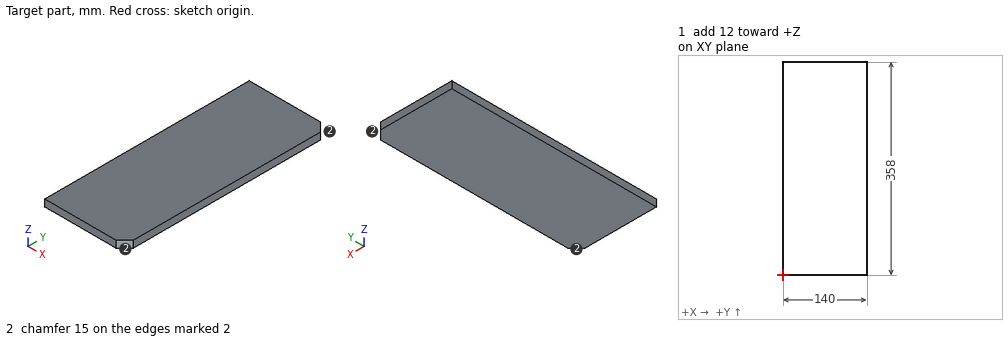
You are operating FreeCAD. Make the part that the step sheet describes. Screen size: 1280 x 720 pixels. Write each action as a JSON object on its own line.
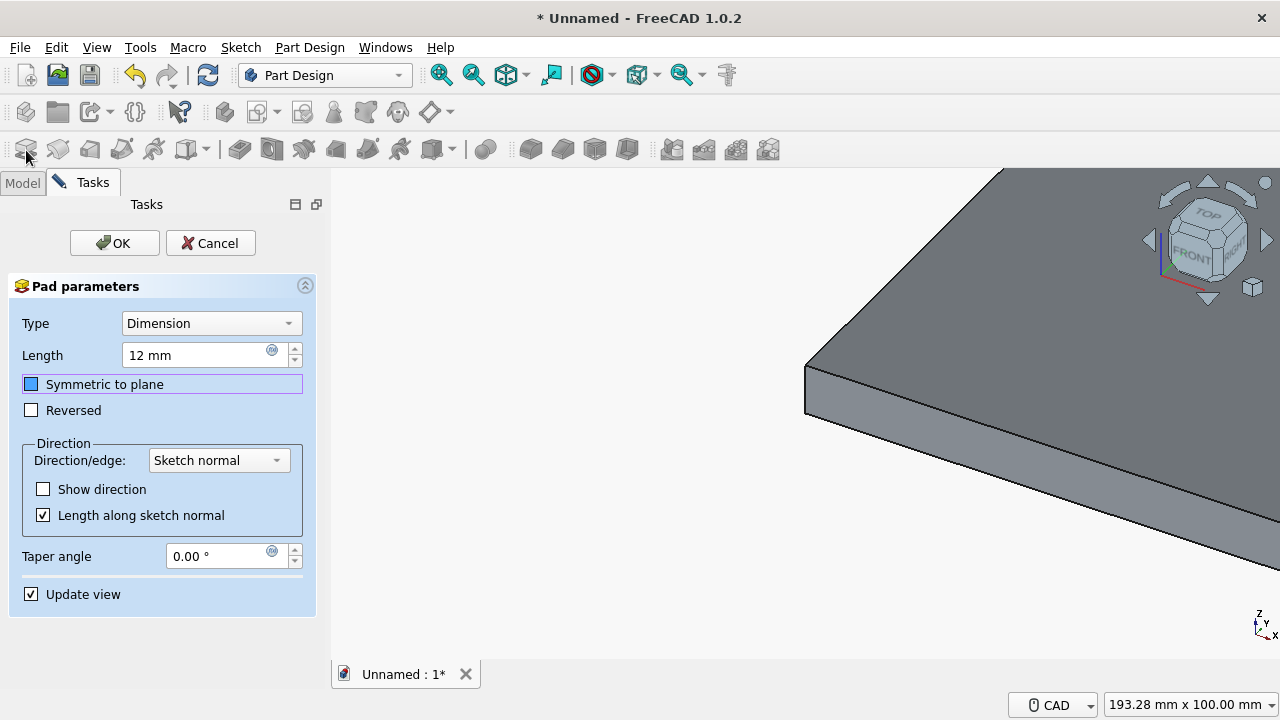
{"action": "left_click", "coordinate": [115, 243]}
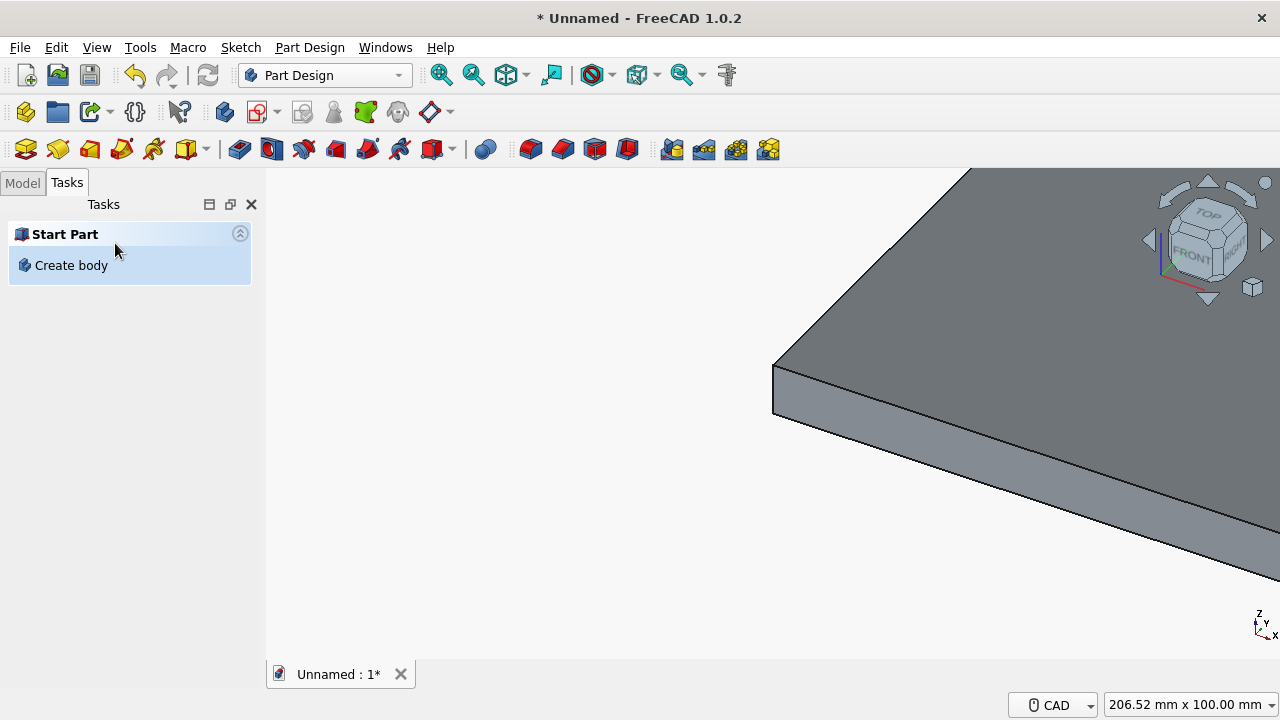
{"action": "left_click", "coordinate": [442, 76]}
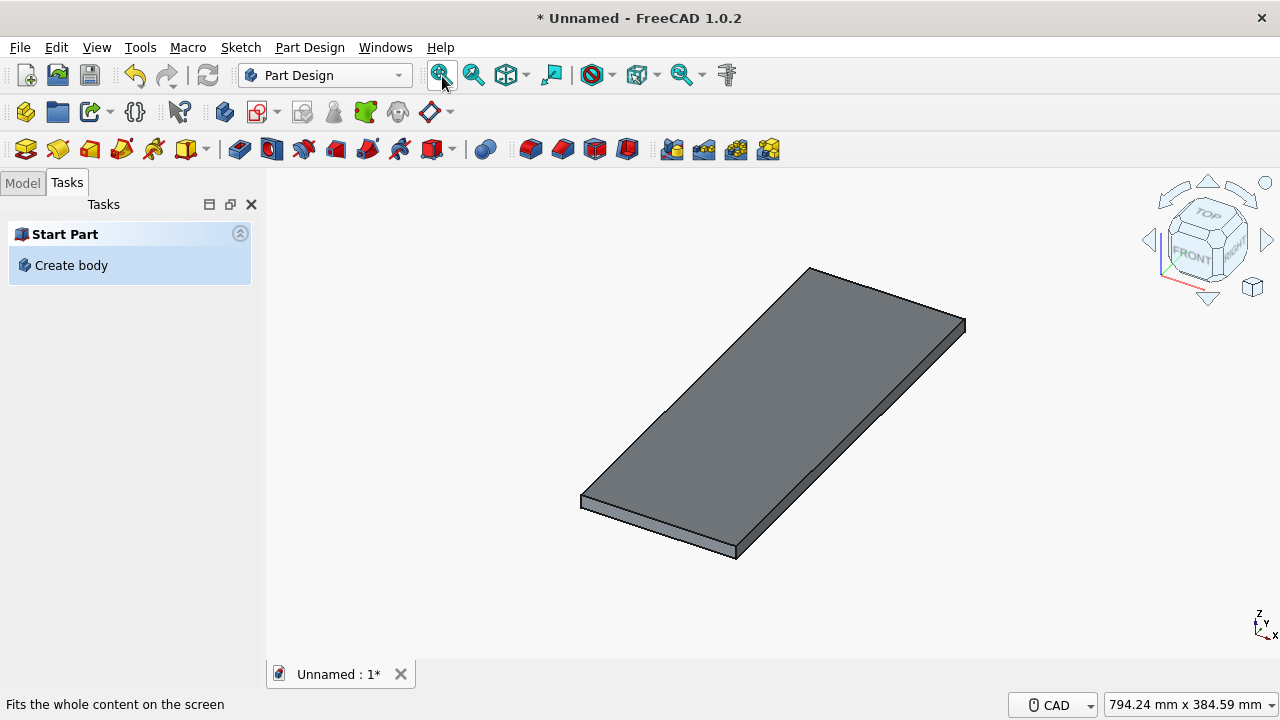
{"action": "left_click", "coordinate": [736, 552]}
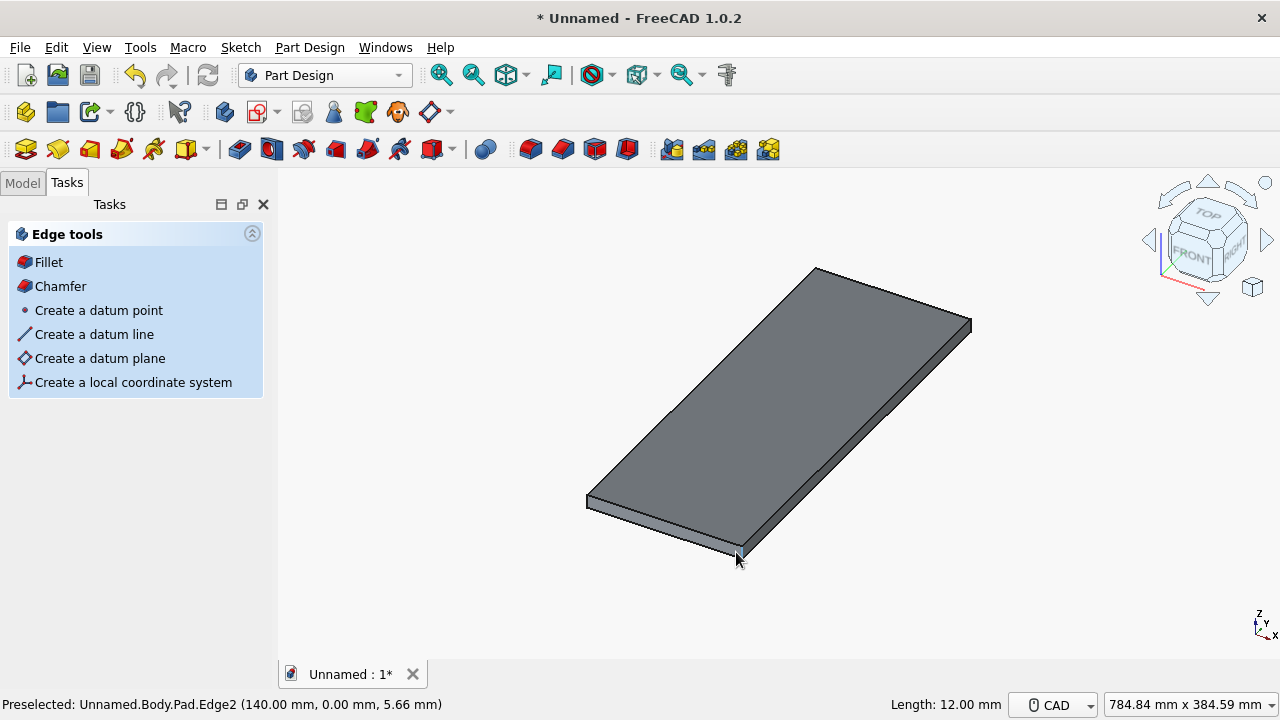
{"action": "scroll", "coordinate": [971, 325], "scroll_direction": "up", "scroll_amount": 5}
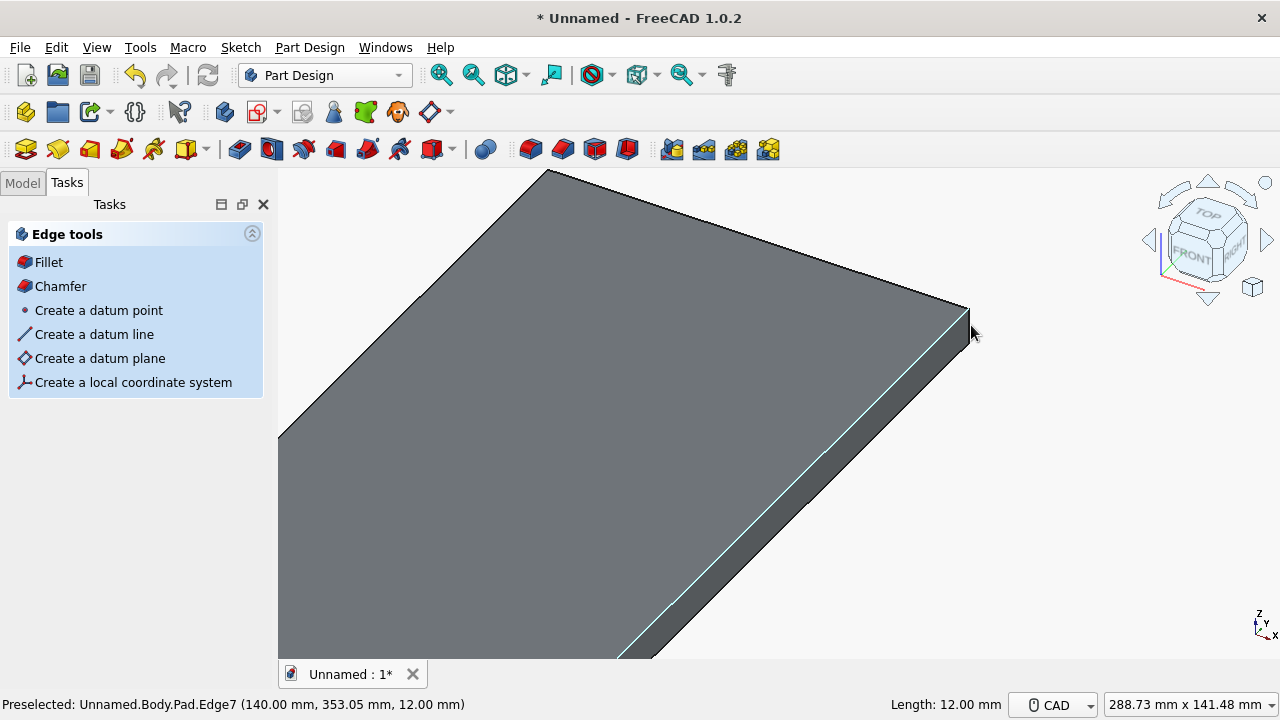
{"action": "left_click", "coordinate": [442, 76]}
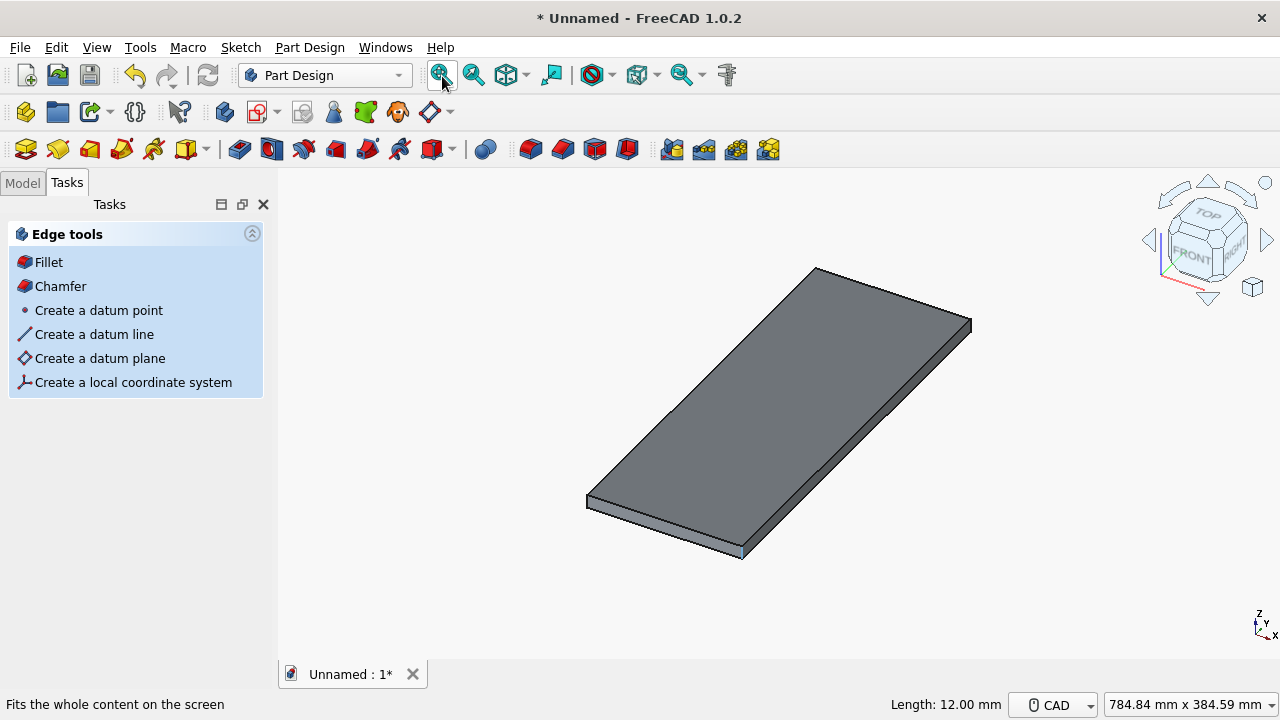
{"action": "key", "text": "0"}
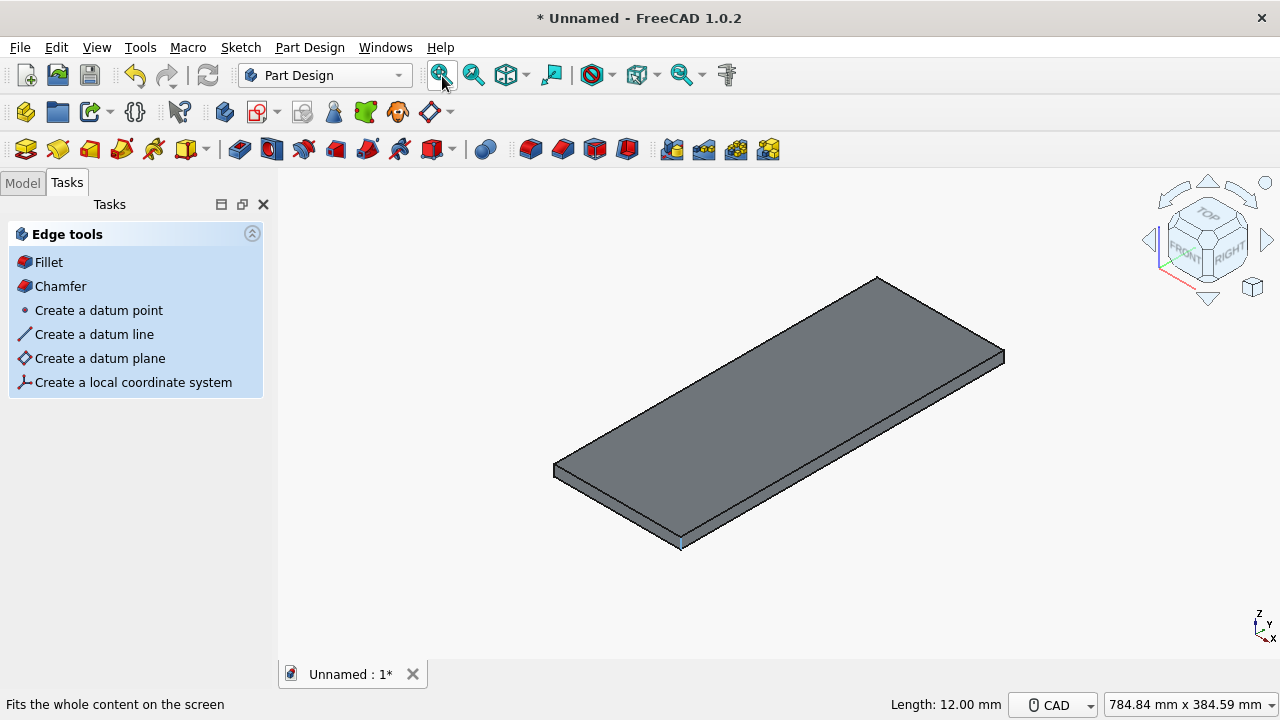
{"action": "scroll", "coordinate": [1004, 356], "scroll_direction": "up", "scroll_amount": 5}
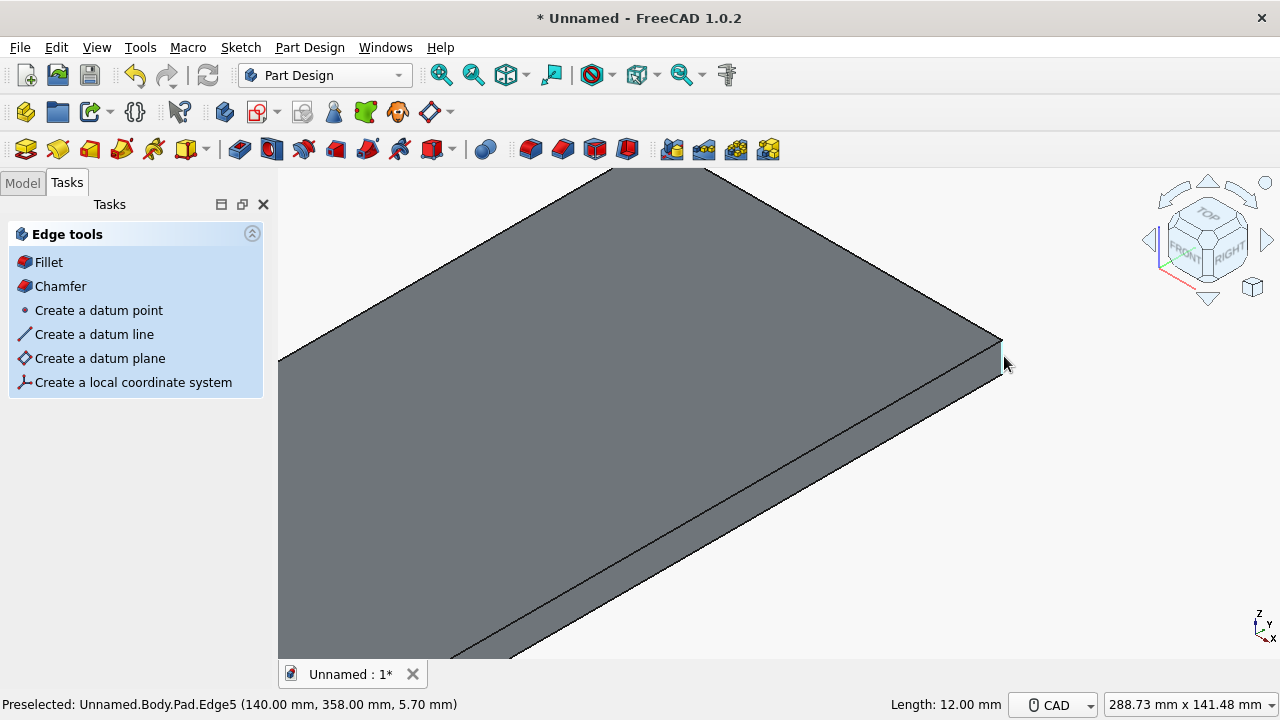
{"action": "key", "text": "v f"}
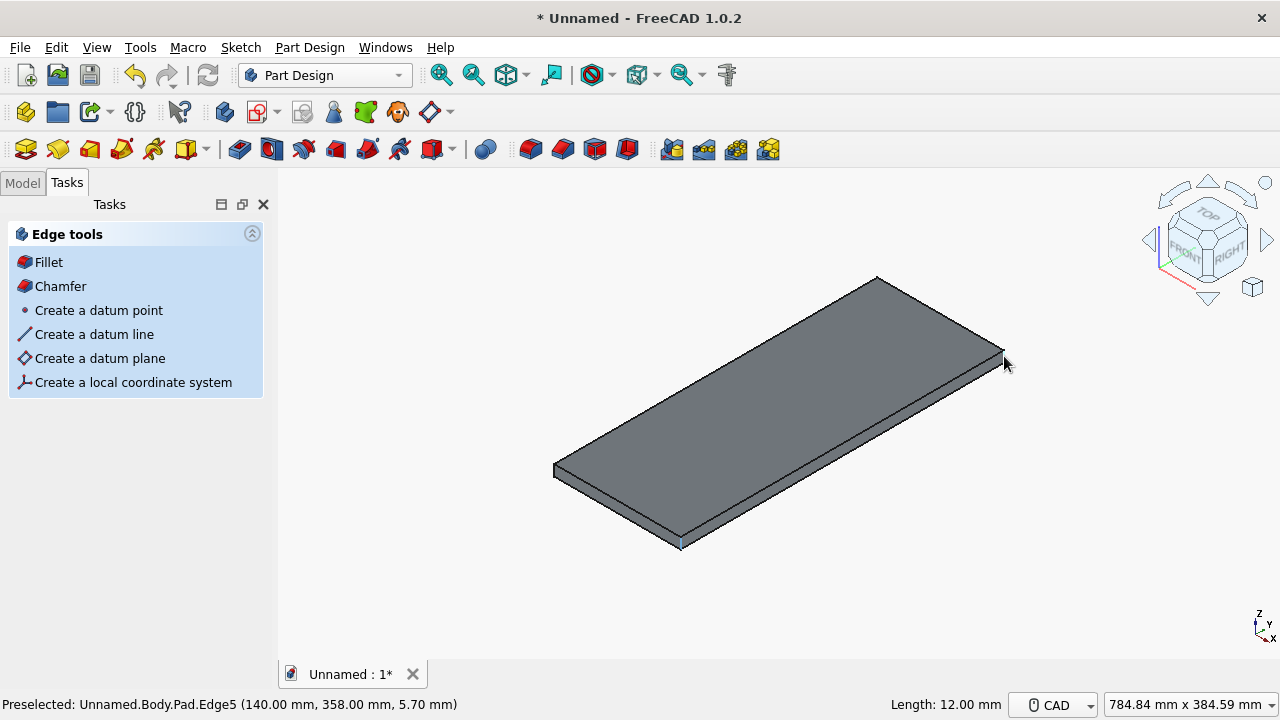
{"action": "key", "text": "2"}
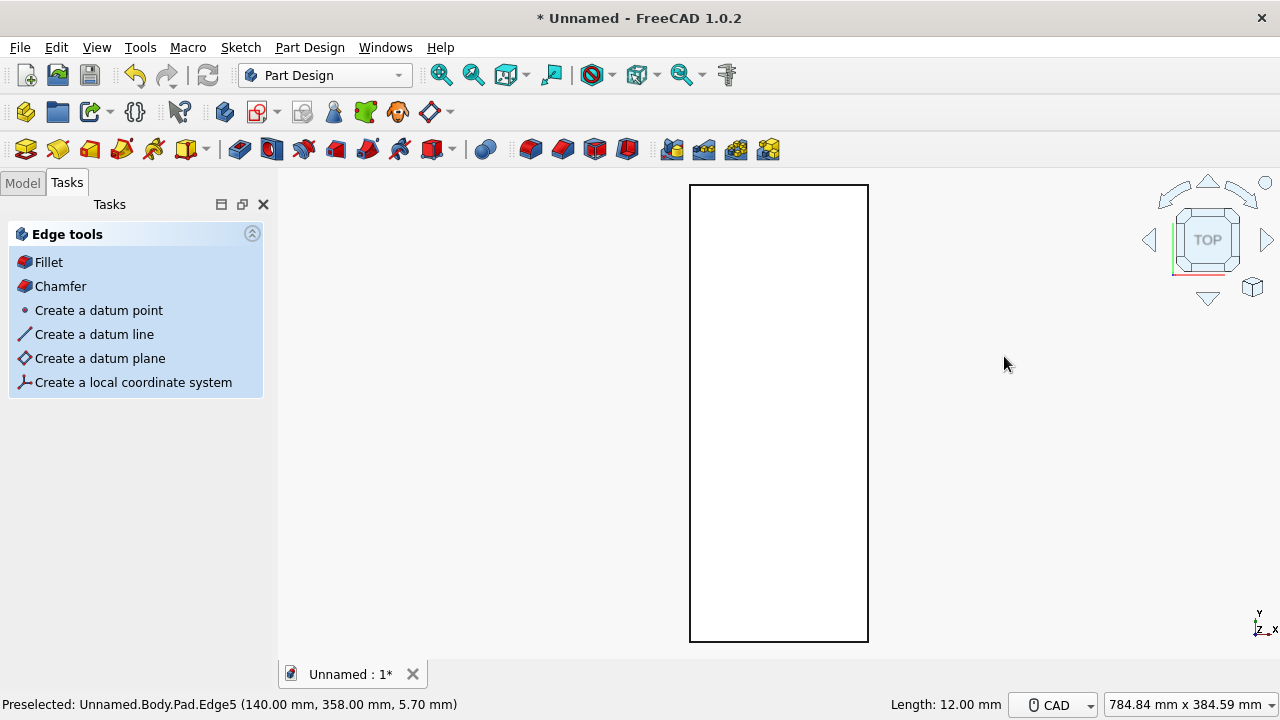
{"action": "key", "text": "1"}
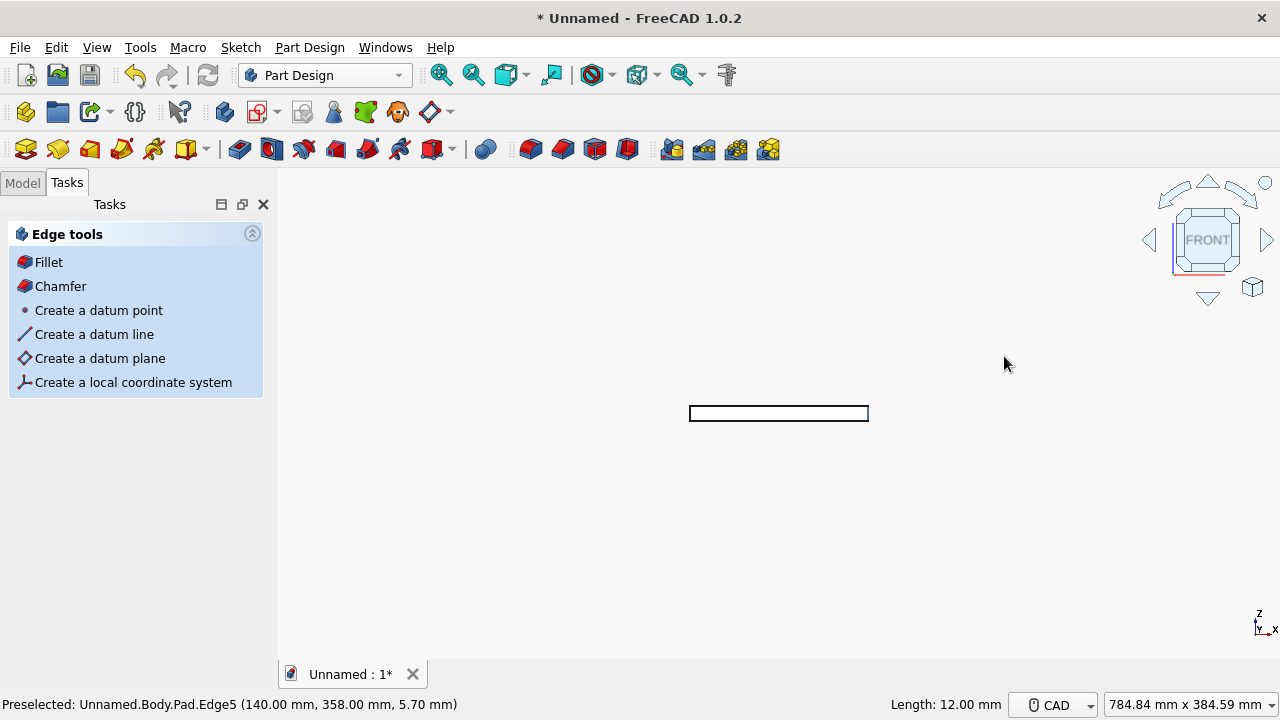
{"action": "key", "text": "v f"}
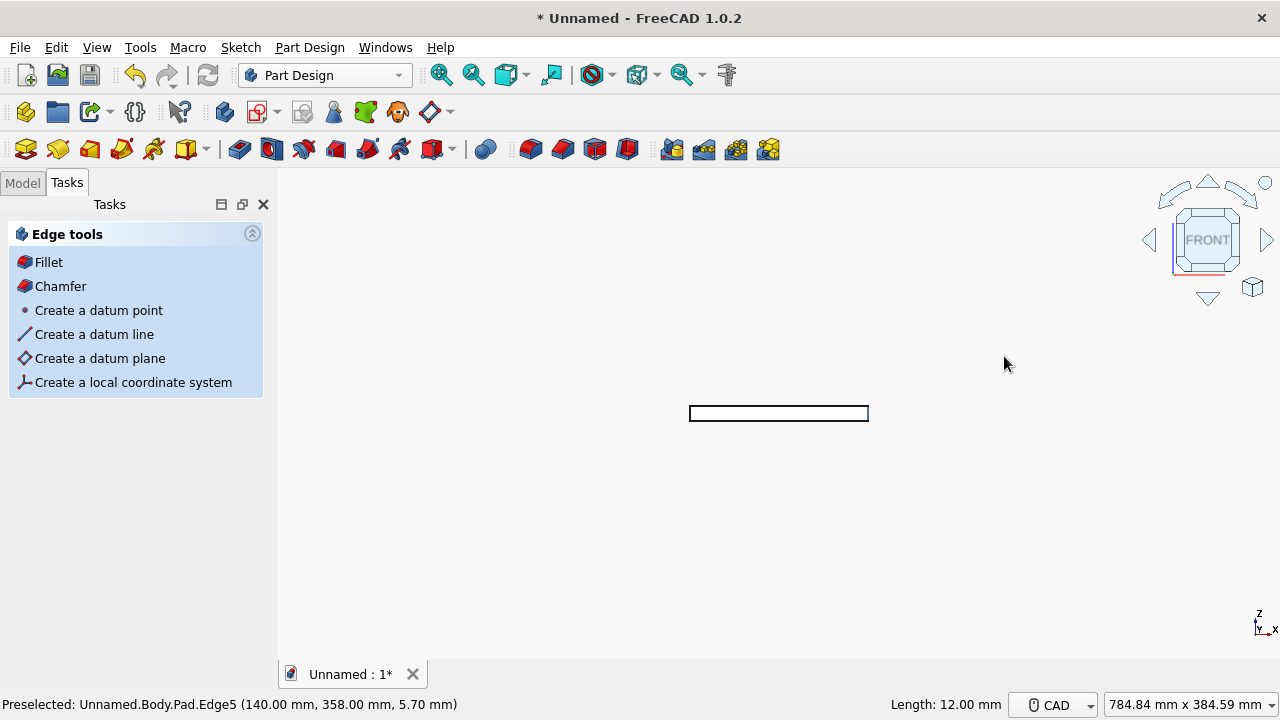
{"action": "scroll", "coordinate": [868, 413], "scroll_direction": "up", "scroll_amount": 5}